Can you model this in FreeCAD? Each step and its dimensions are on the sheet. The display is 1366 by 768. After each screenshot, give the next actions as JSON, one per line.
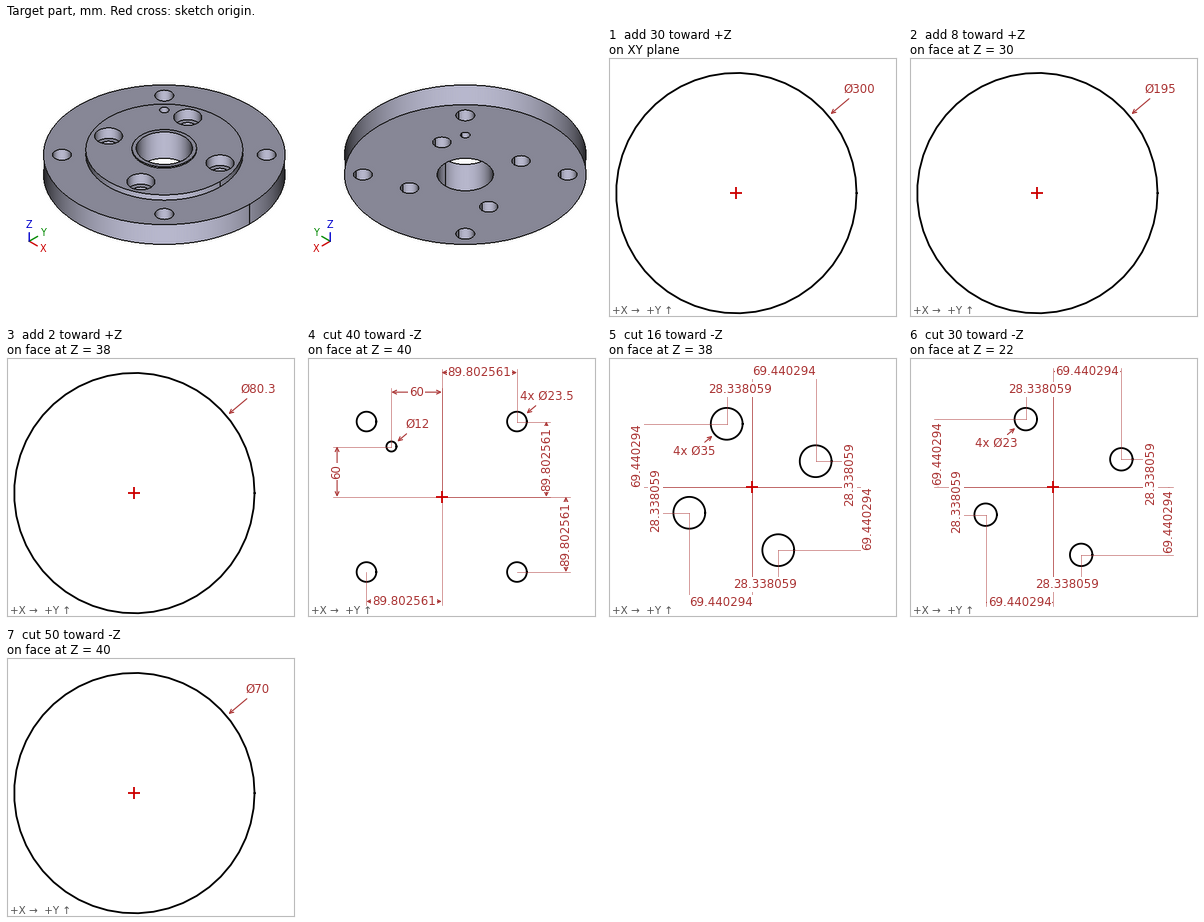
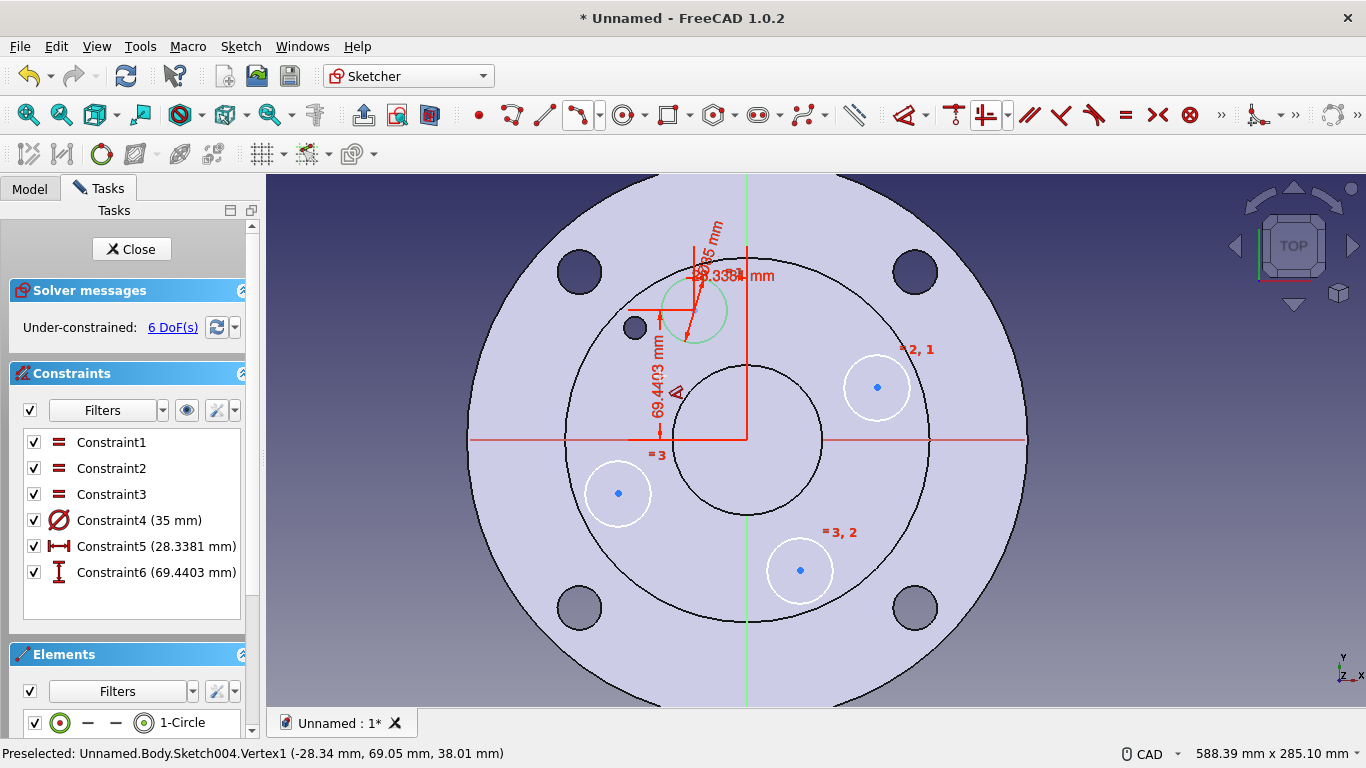
{"action": "left_click", "coordinate": [877, 388]}
{"action": "left_click", "coordinate": [812, 354]}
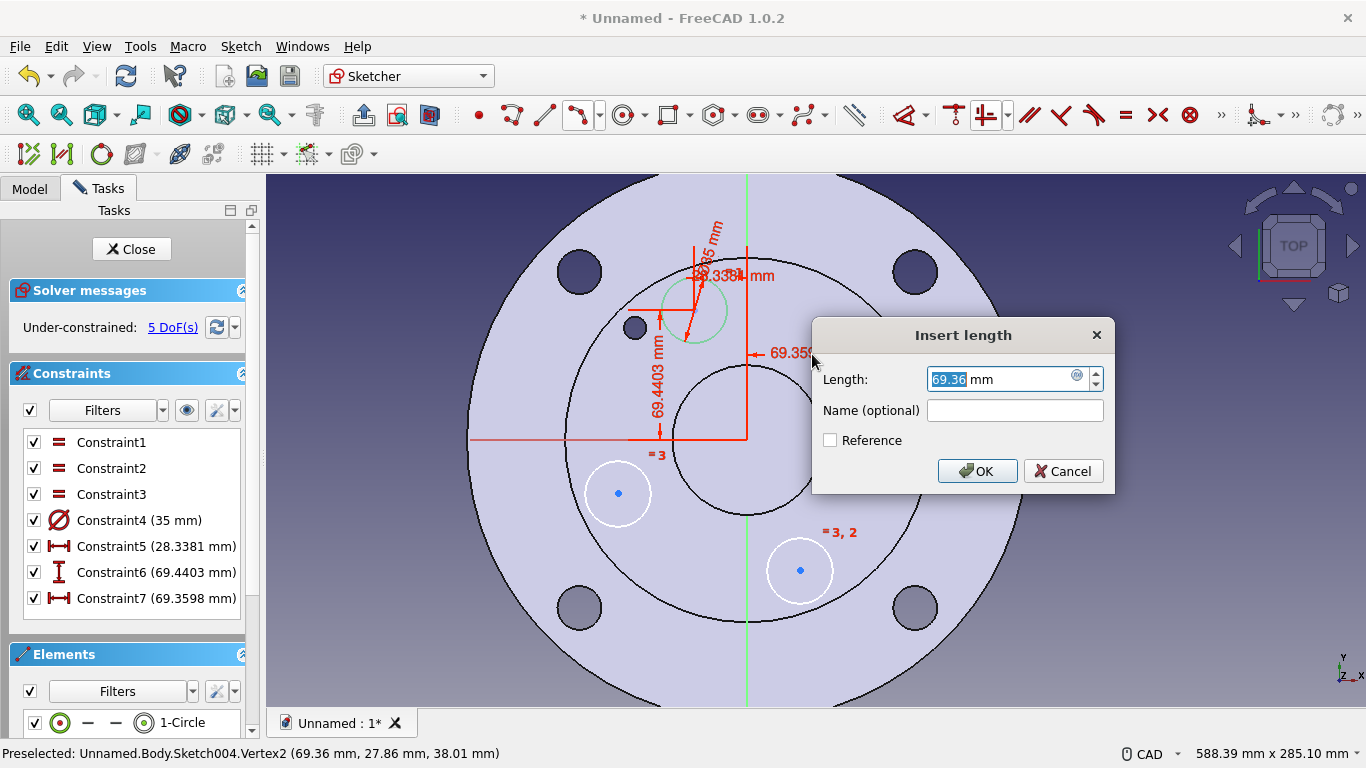
{"action": "type", "text": "69.440294"}
{"action": "key", "text": "Return"}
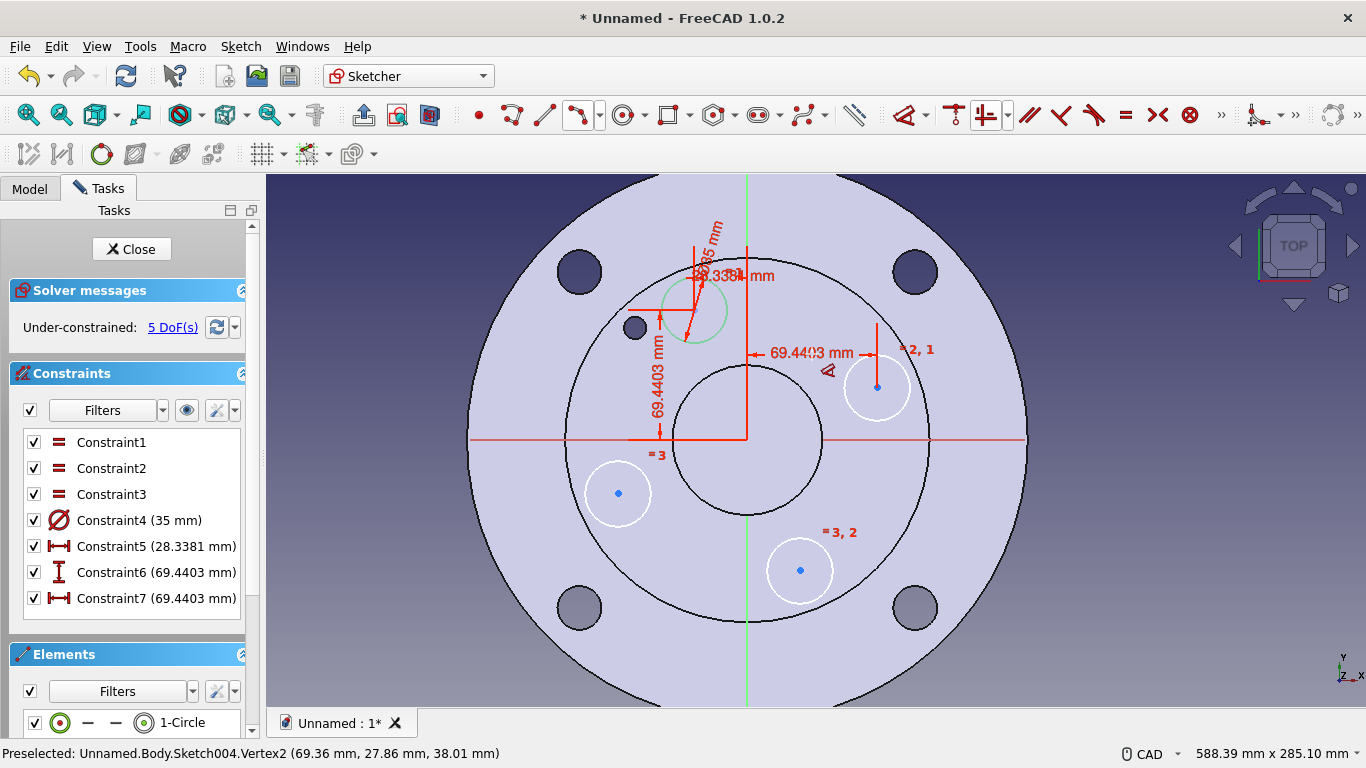
{"action": "left_click", "coordinate": [877, 388]}
{"action": "left_click", "coordinate": [911, 426]}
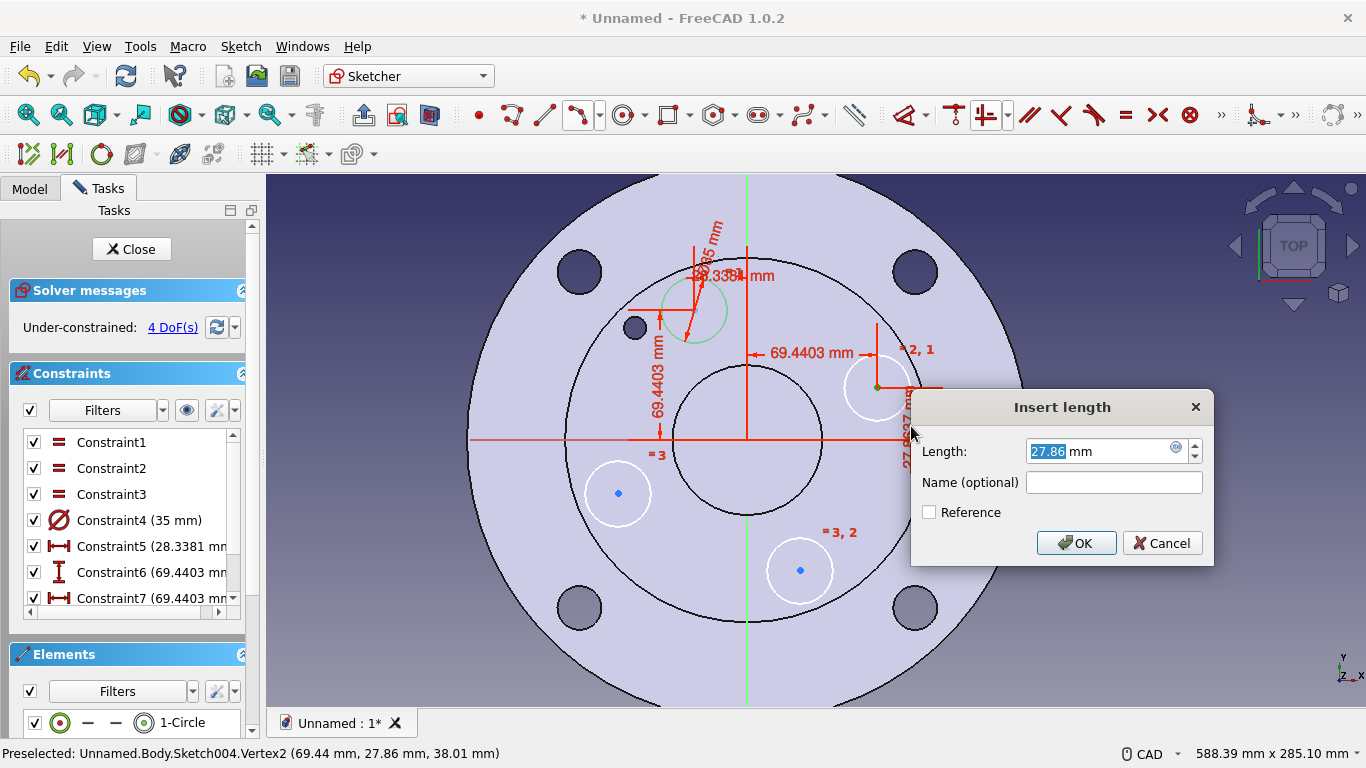
{"action": "type", "text": "28.338059"}
{"action": "key", "text": "Return"}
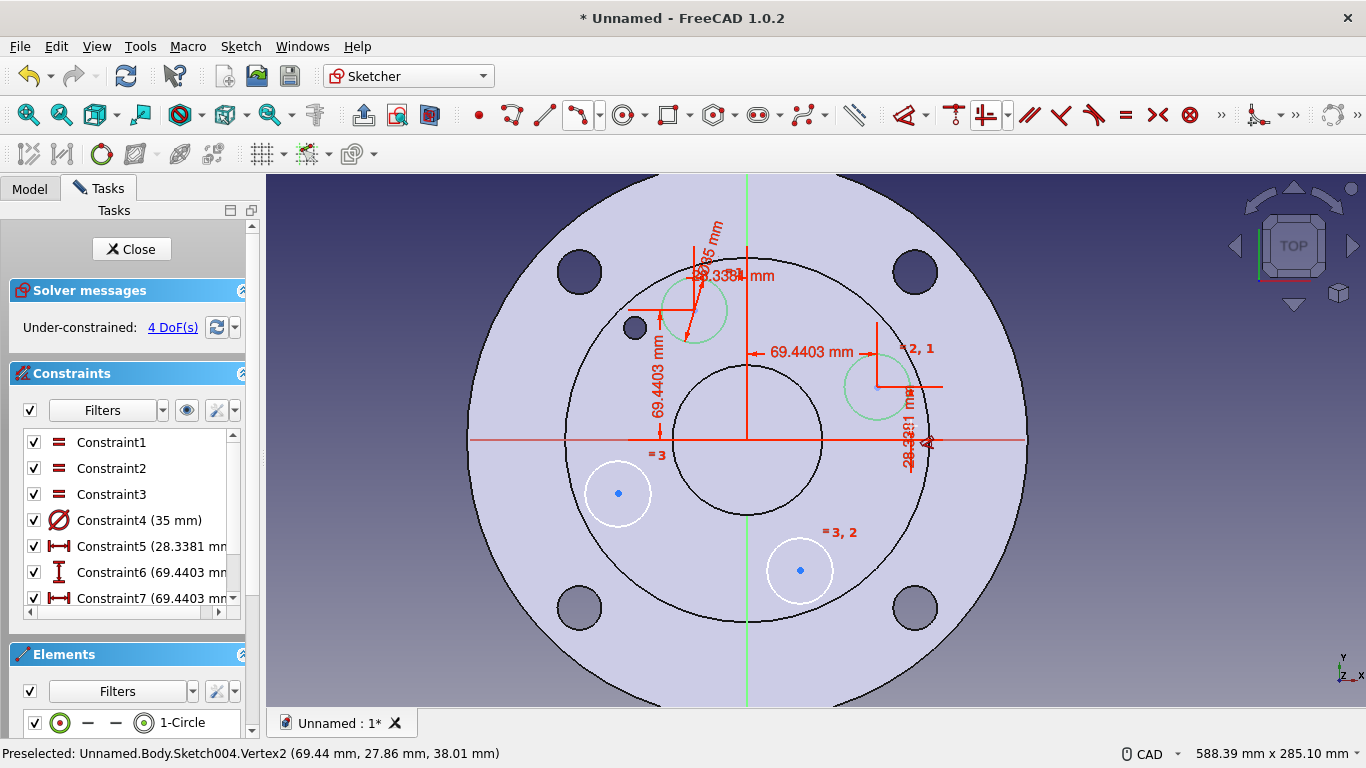
{"action": "left_click", "coordinate": [800, 571]}
{"action": "left_click", "coordinate": [762, 605]}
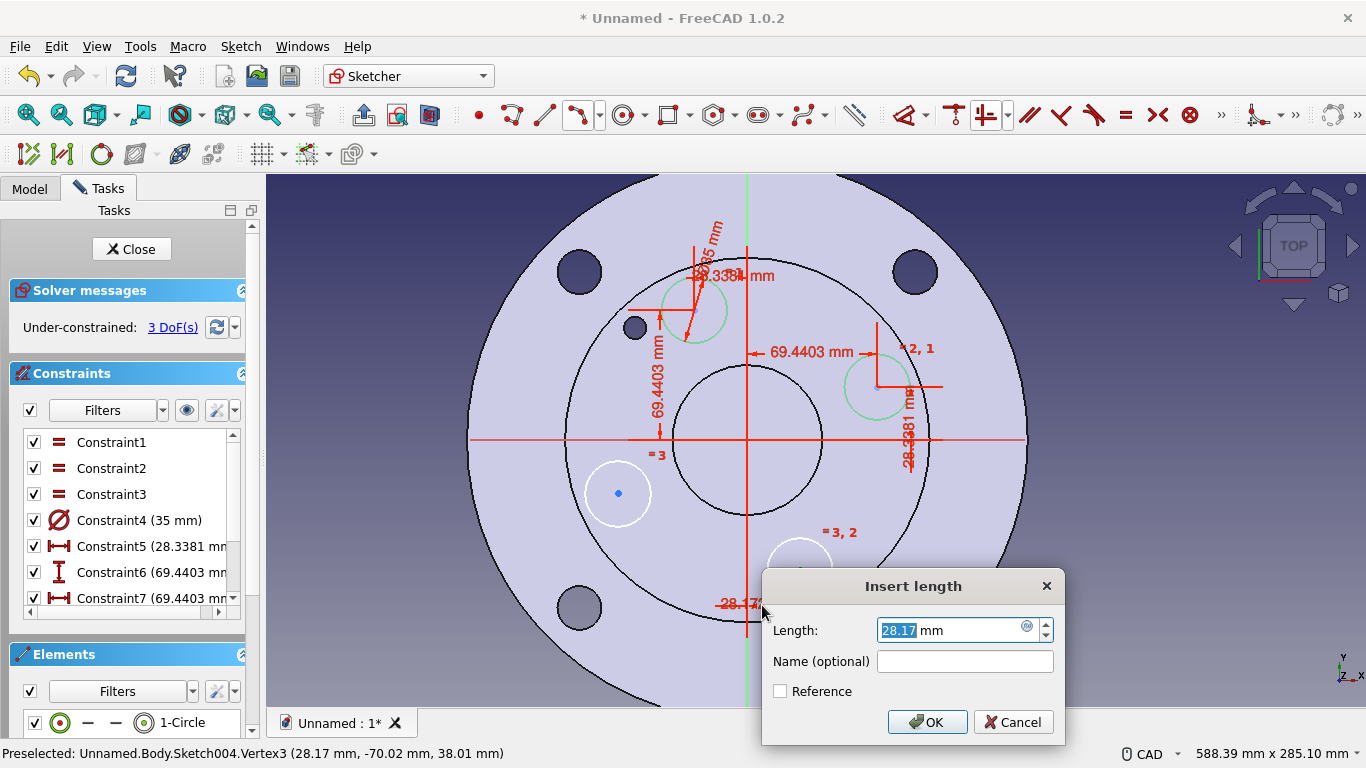
{"action": "type", "text": "28.338059"}
{"action": "key", "text": "Return"}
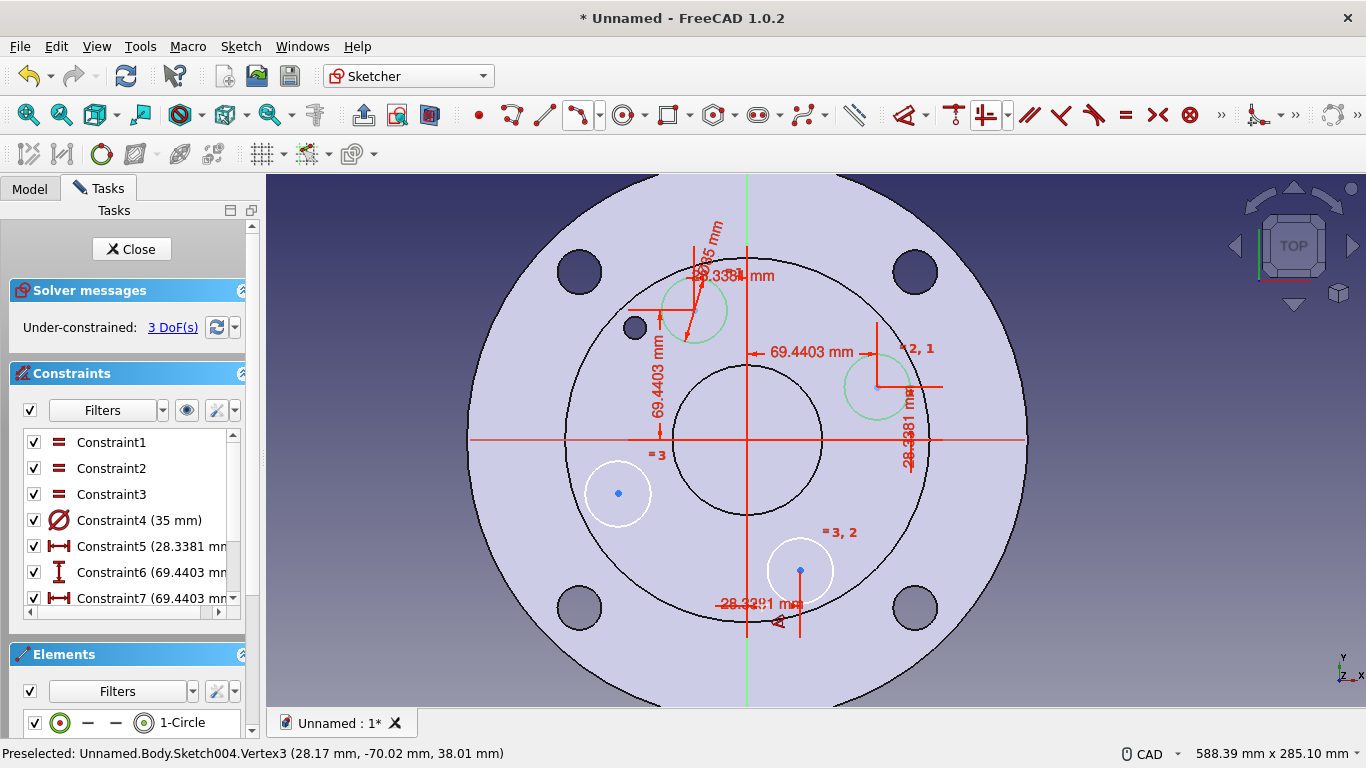
{"action": "left_click", "coordinate": [800, 571]}
{"action": "left_click", "coordinate": [834, 506]}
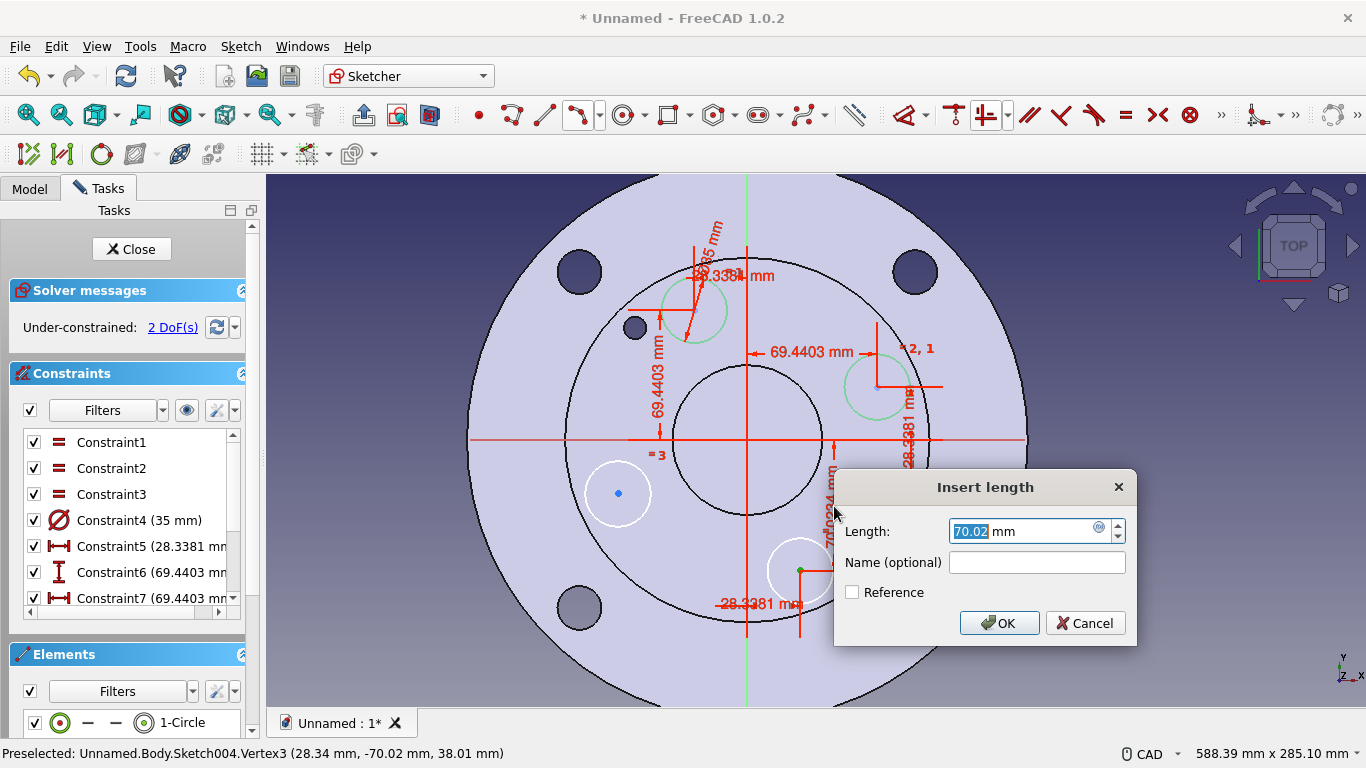
{"action": "type", "text": "69.440294"}
{"action": "key", "text": "Return"}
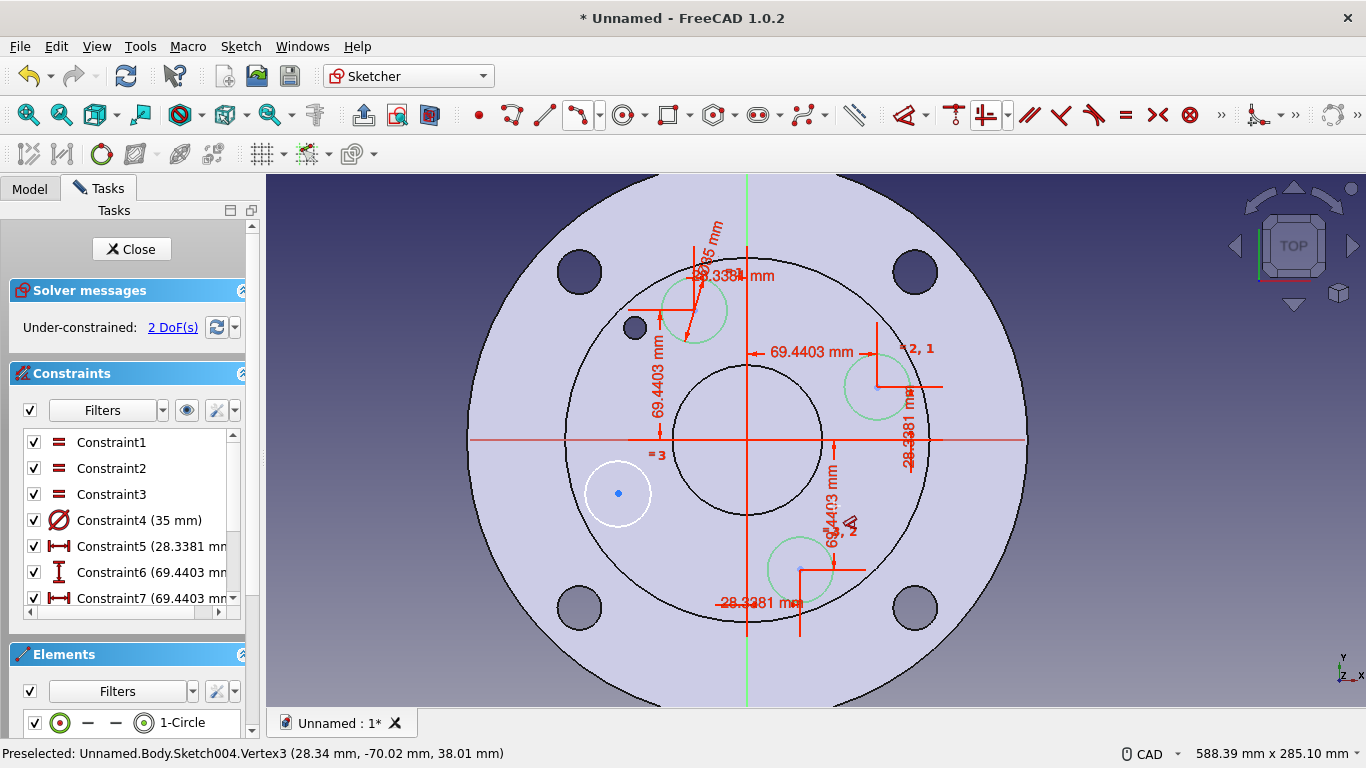
{"action": "left_click", "coordinate": [618, 494]}
{"action": "left_click", "coordinate": [683, 528]}